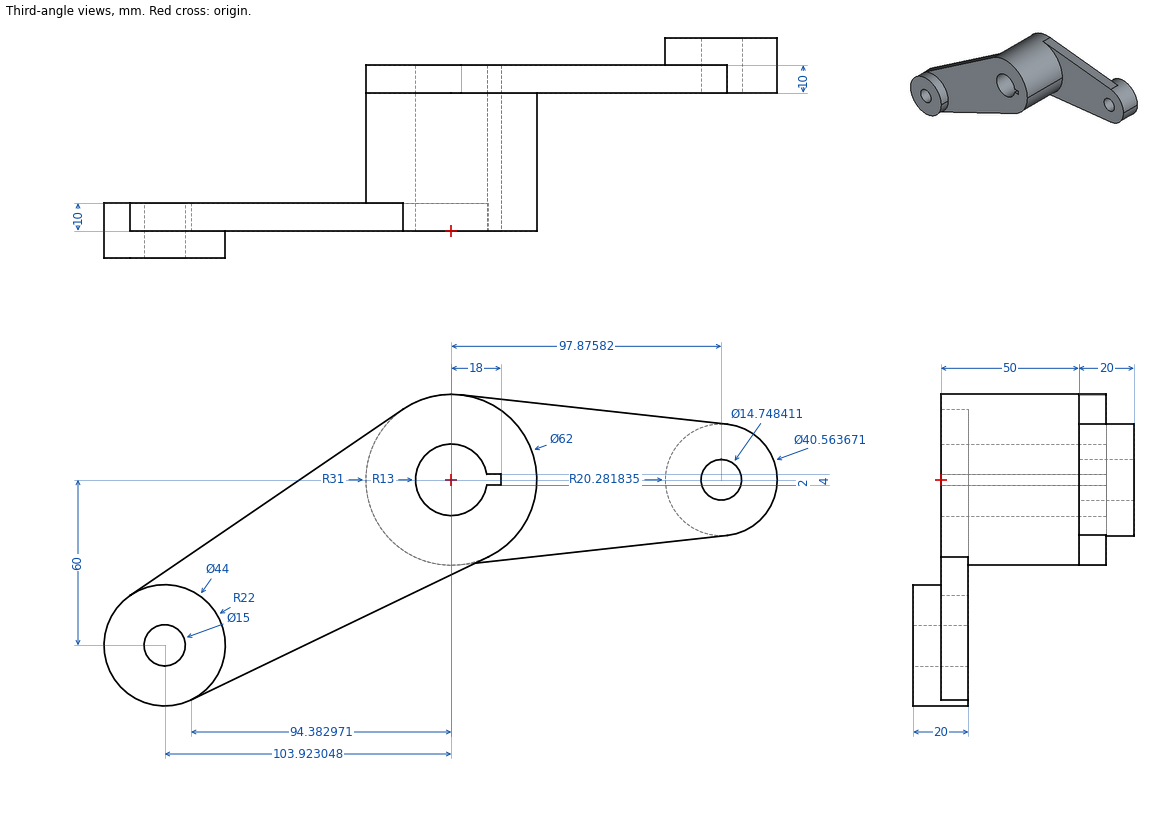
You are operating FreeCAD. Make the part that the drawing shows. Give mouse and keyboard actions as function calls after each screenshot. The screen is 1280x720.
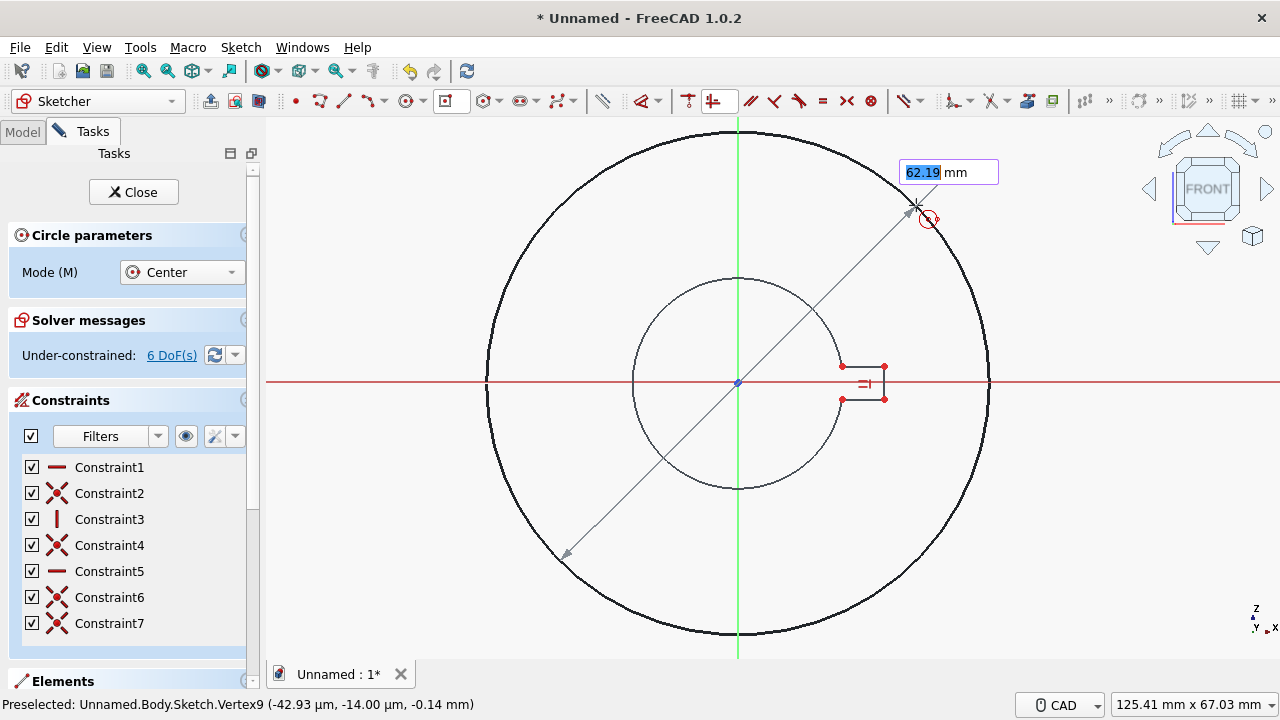
text(62)
key(Return)
key(Escape)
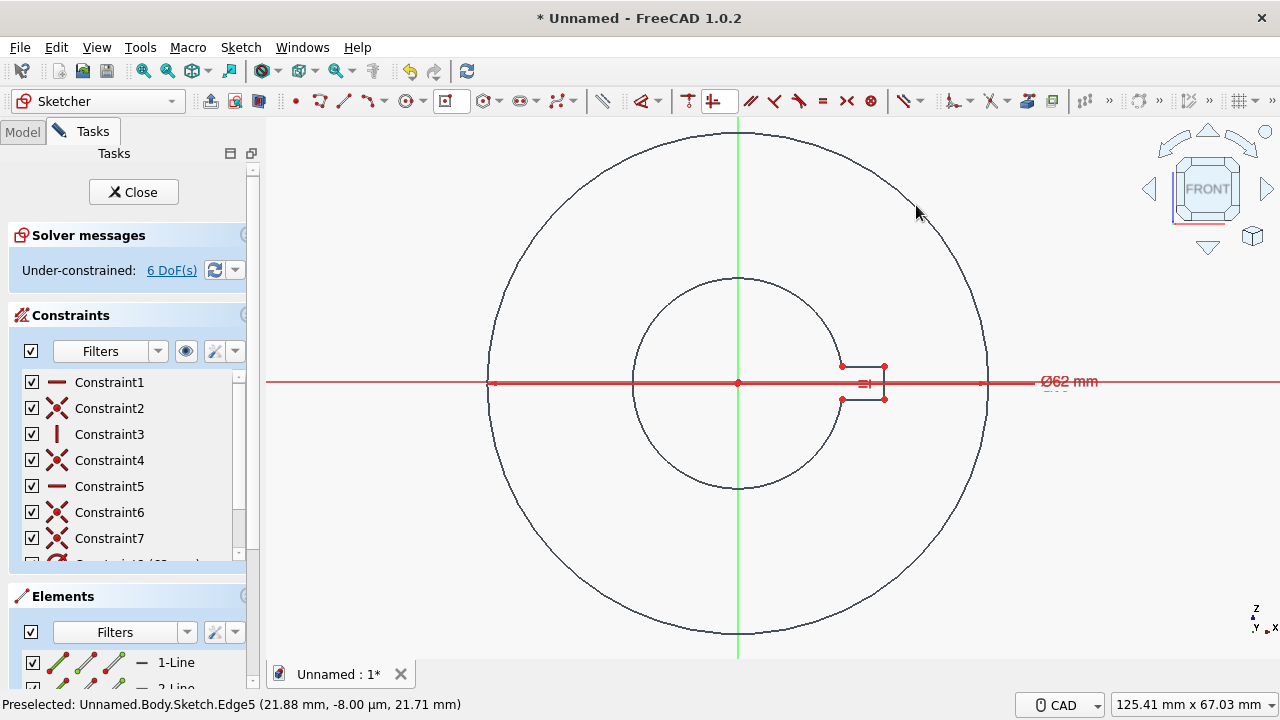
drag(728, 372, 748, 393)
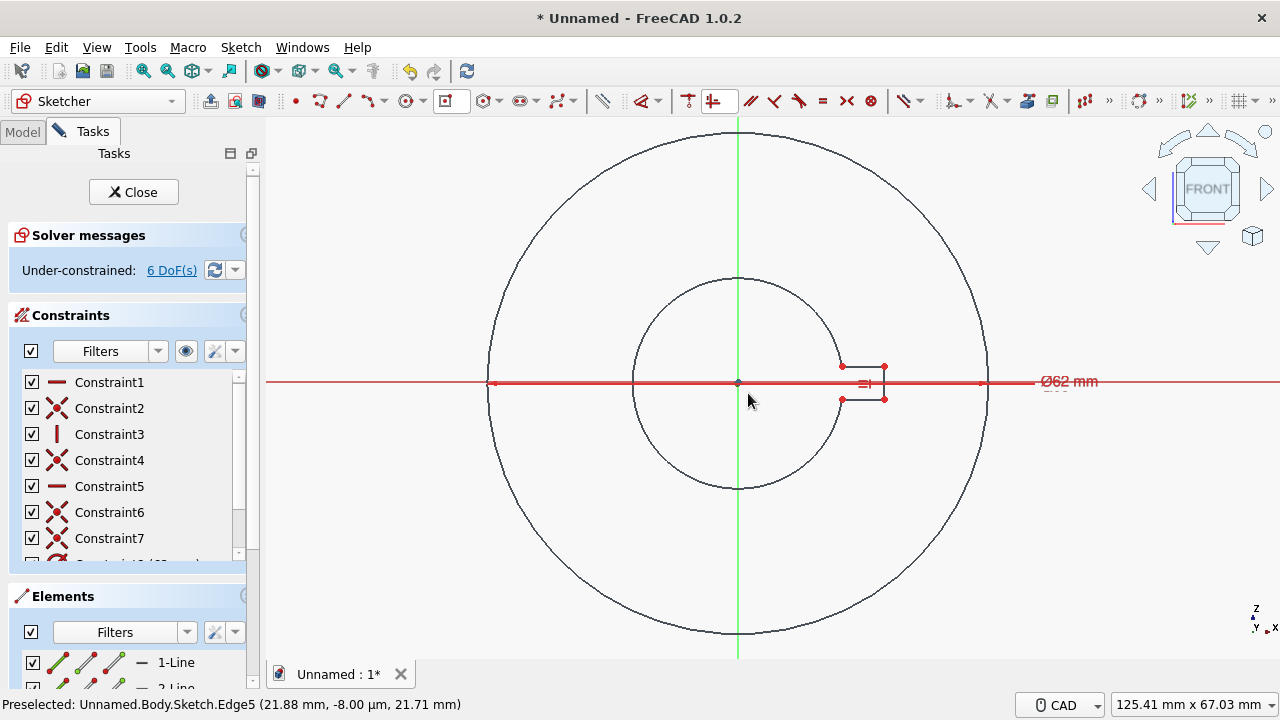
click(688, 102)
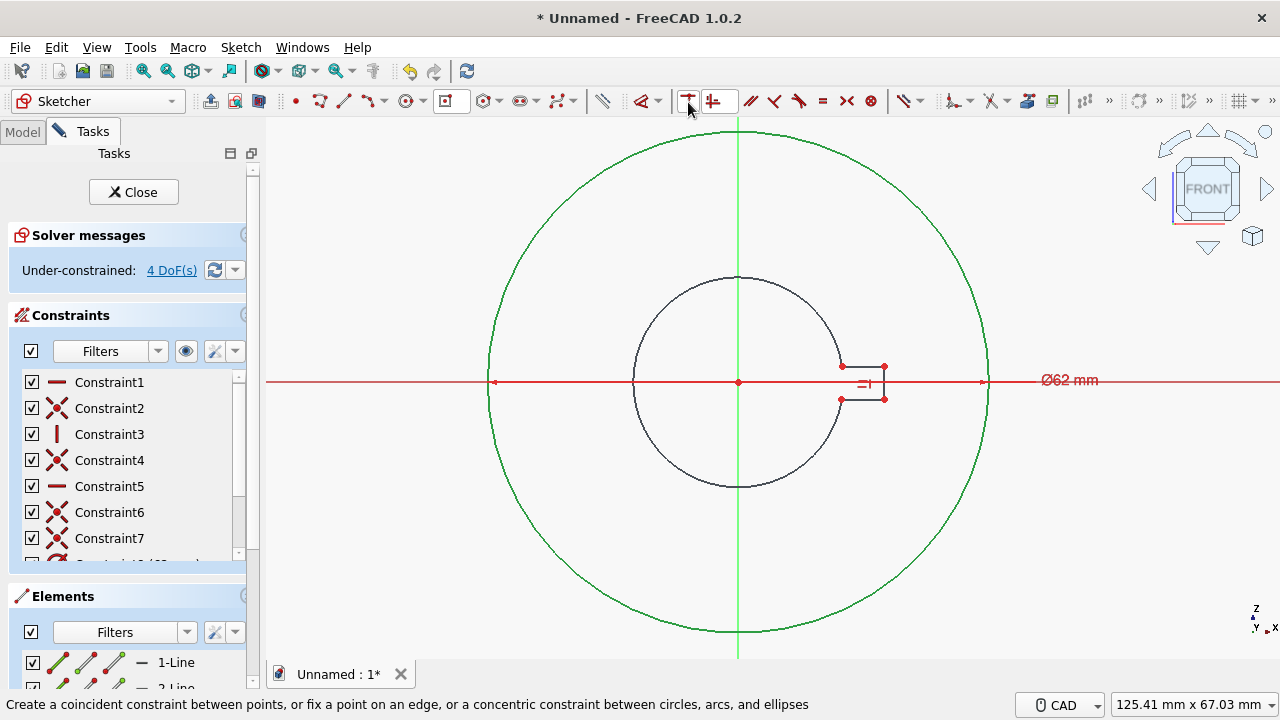
key(d)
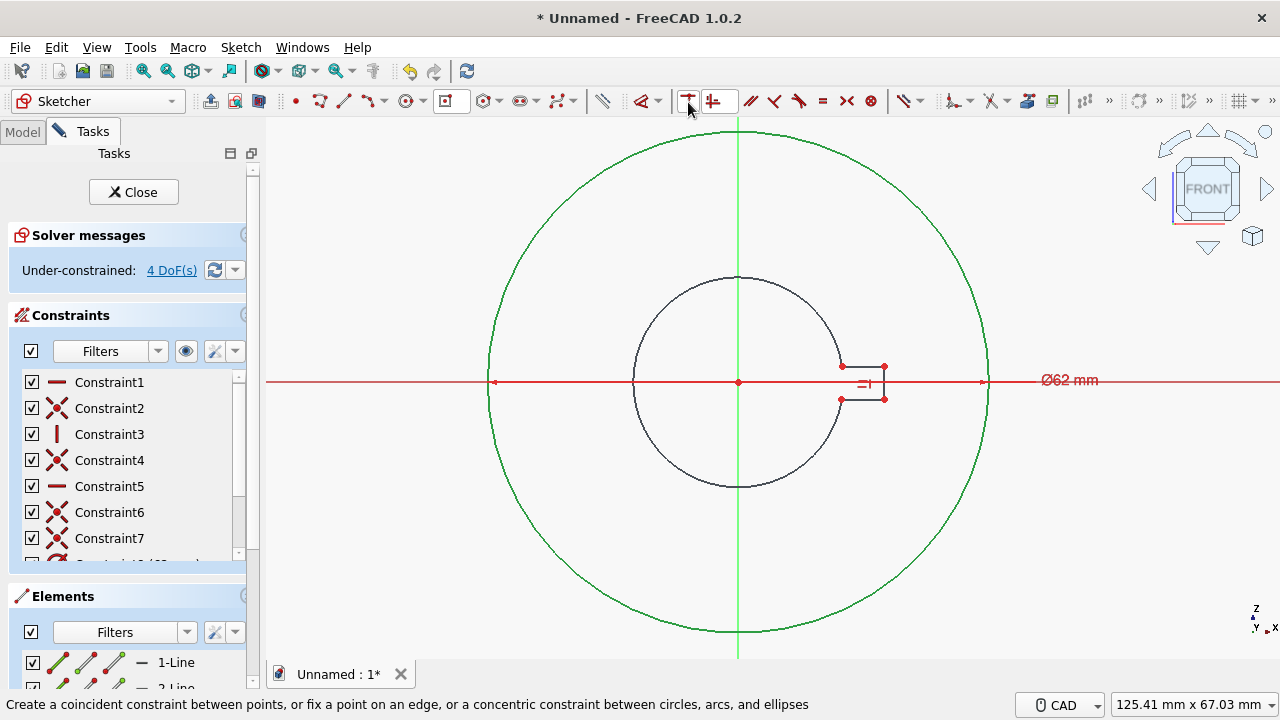
click(701, 284)
click(690, 254)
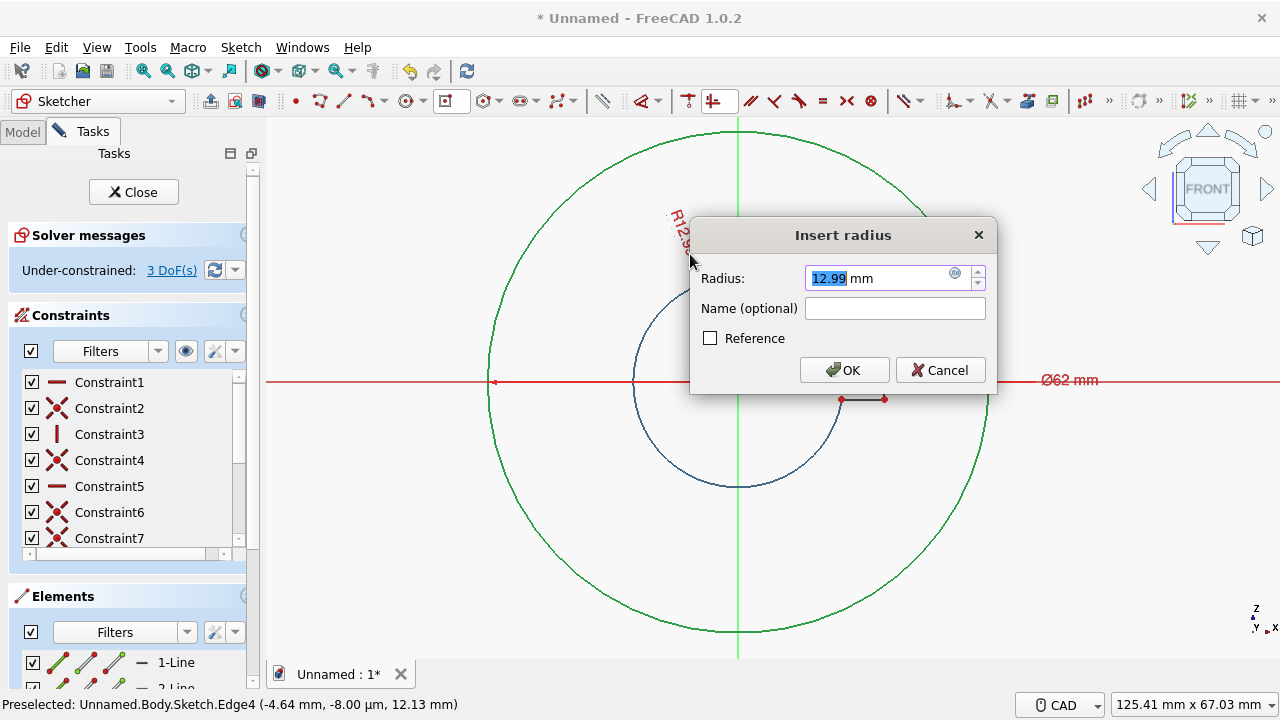
text(13)
key(Return)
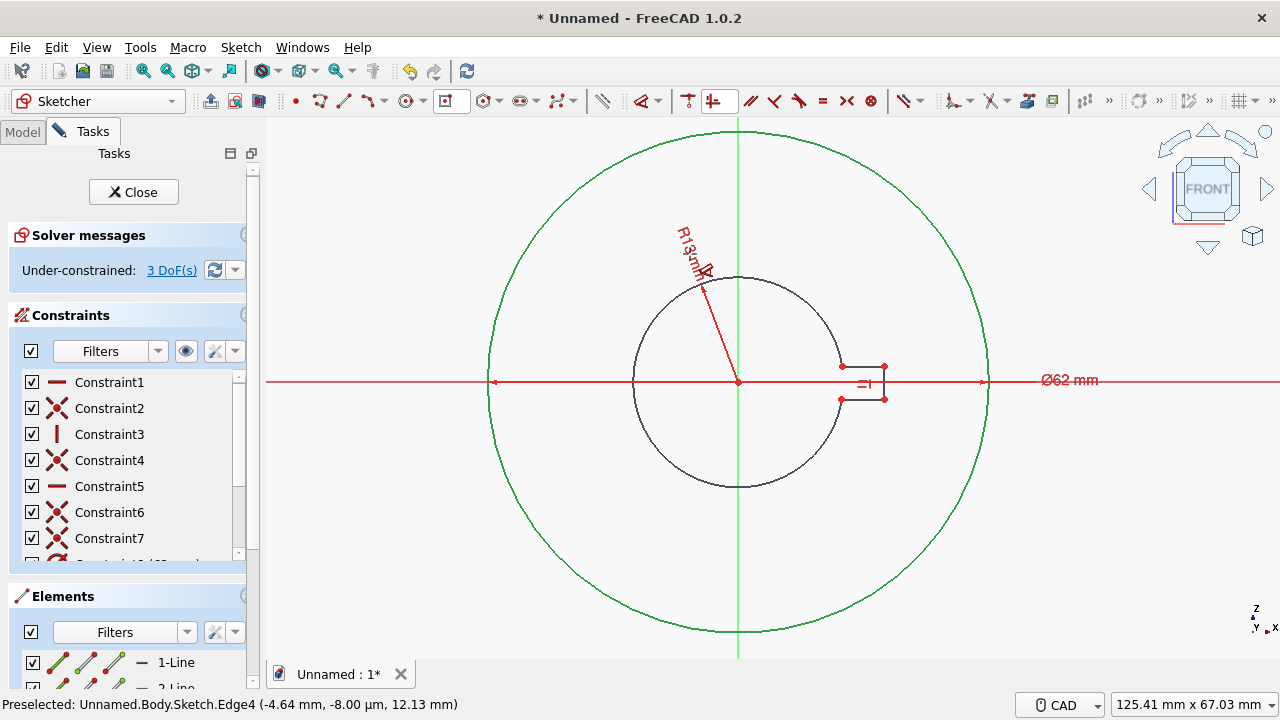
scroll(884, 380, up, 2)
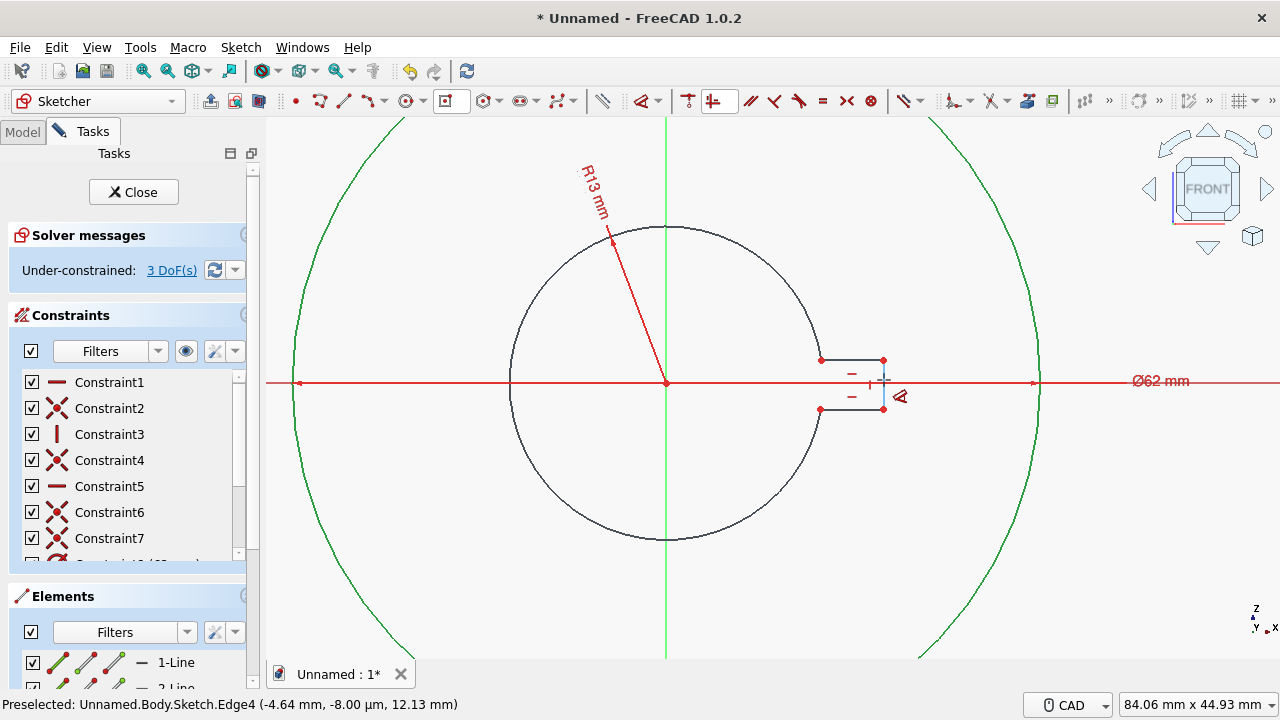
click(884, 380)
click(918, 396)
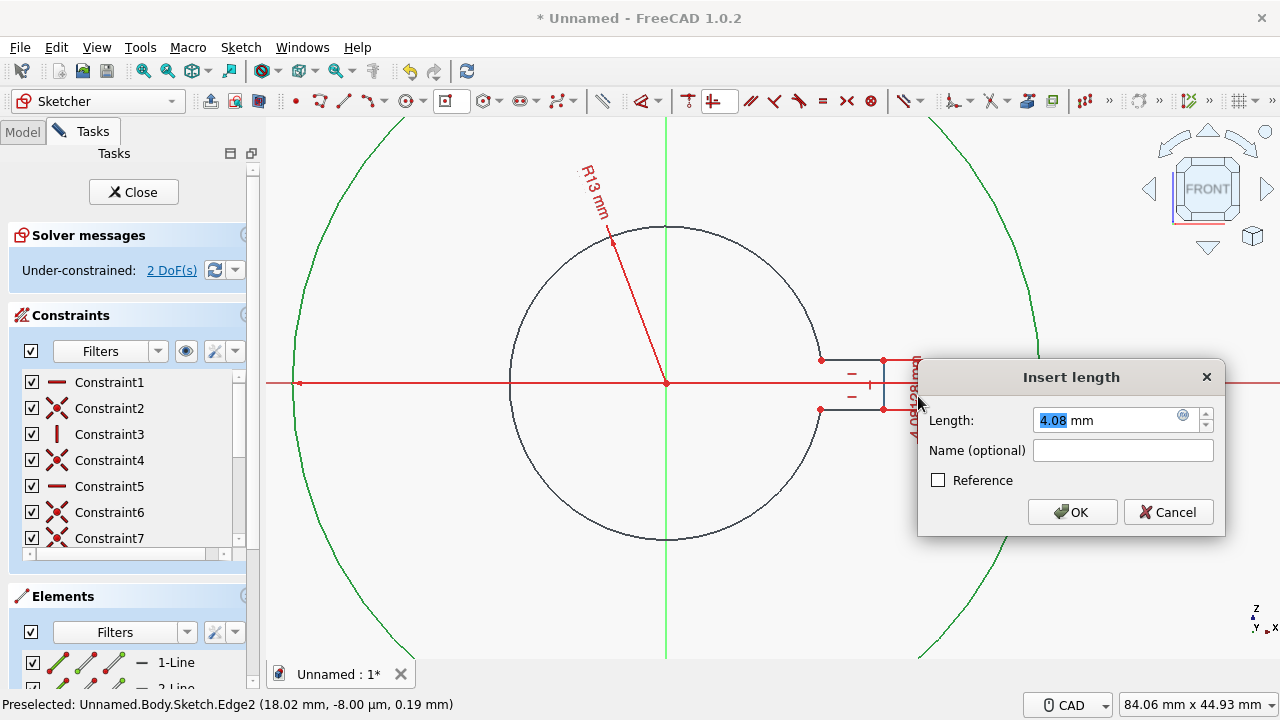
text(4)
key(Return)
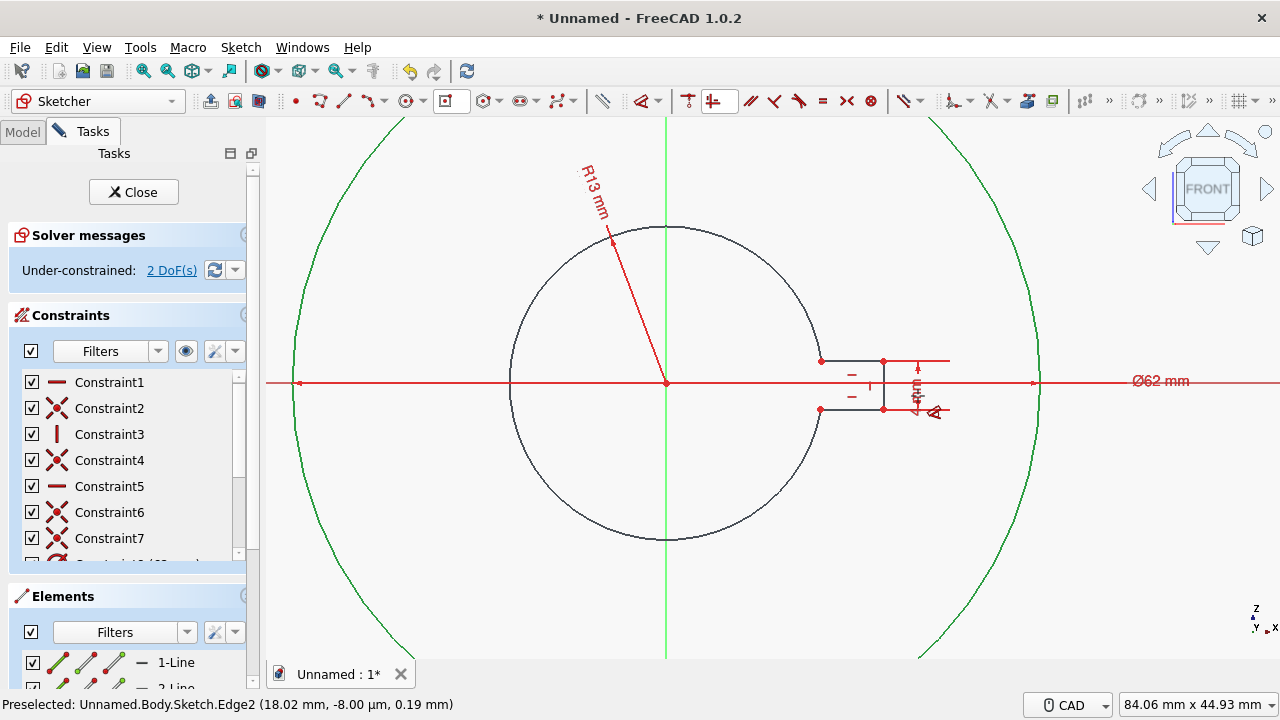
scroll(821, 410, up, 3)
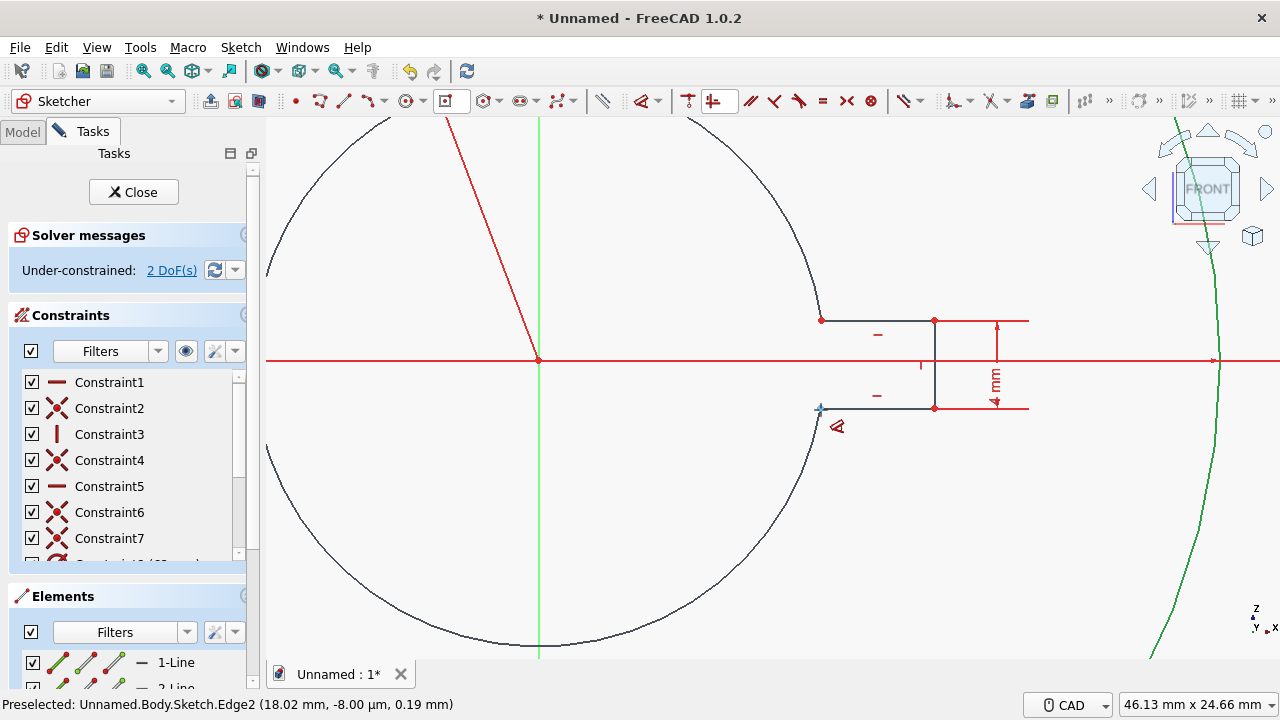
click(820, 409)
click(854, 385)